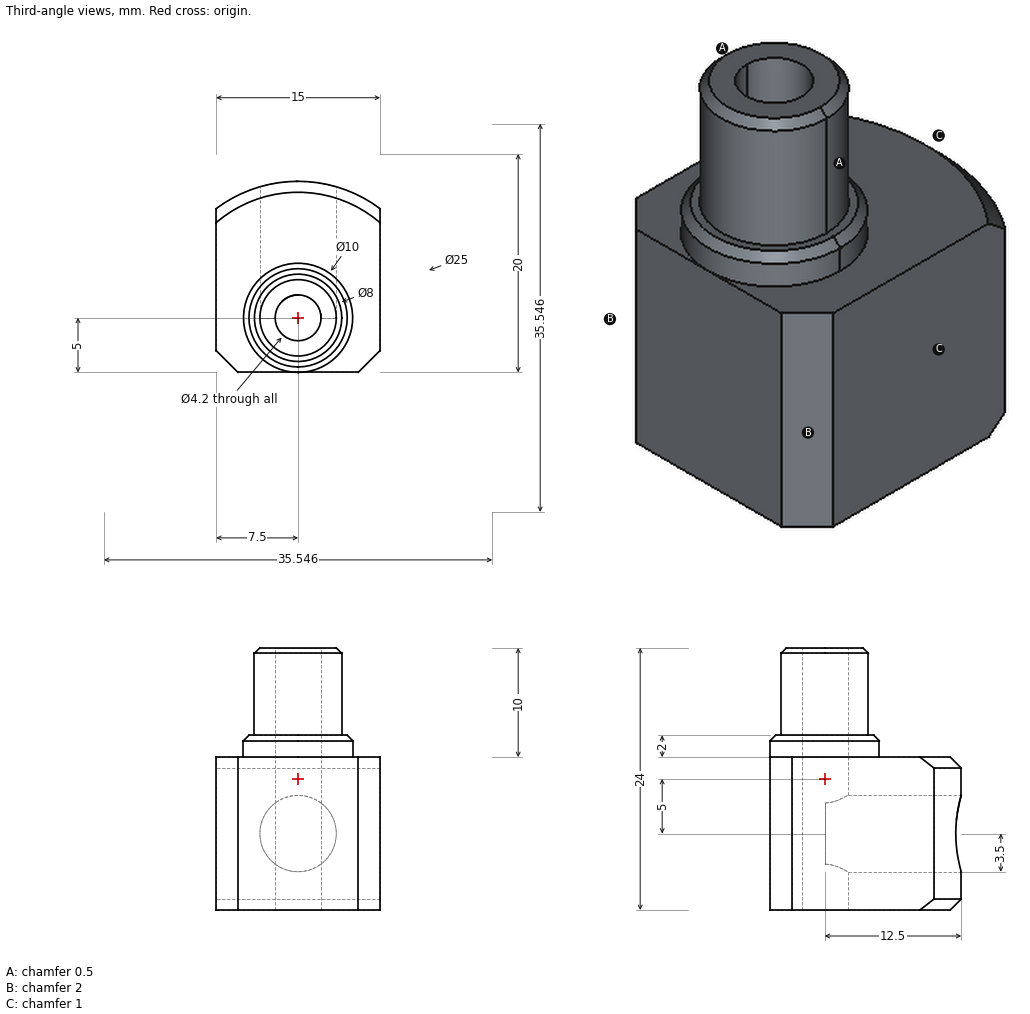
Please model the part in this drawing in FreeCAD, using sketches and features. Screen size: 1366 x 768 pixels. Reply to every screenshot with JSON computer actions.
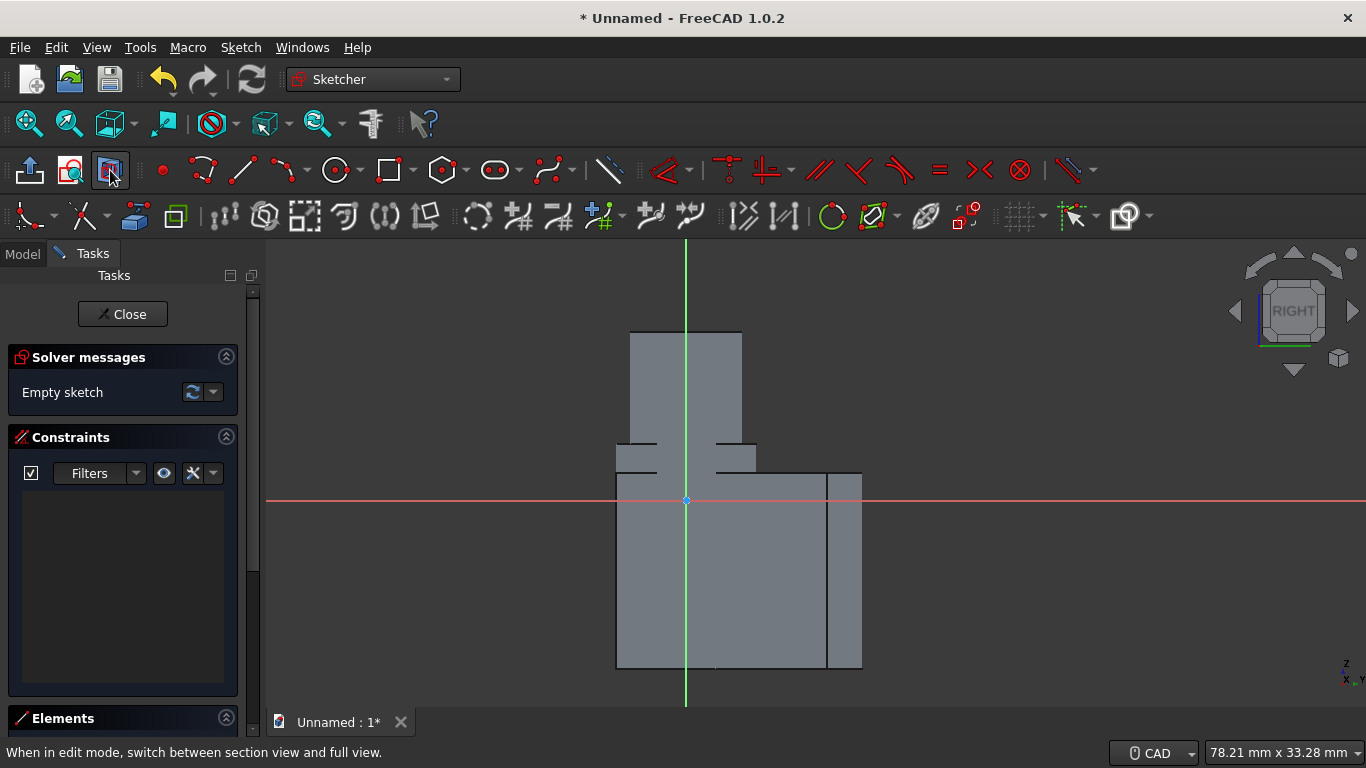
{"action": "scroll", "coordinate": [860, 632], "scroll_direction": "up", "scroll_amount": 4}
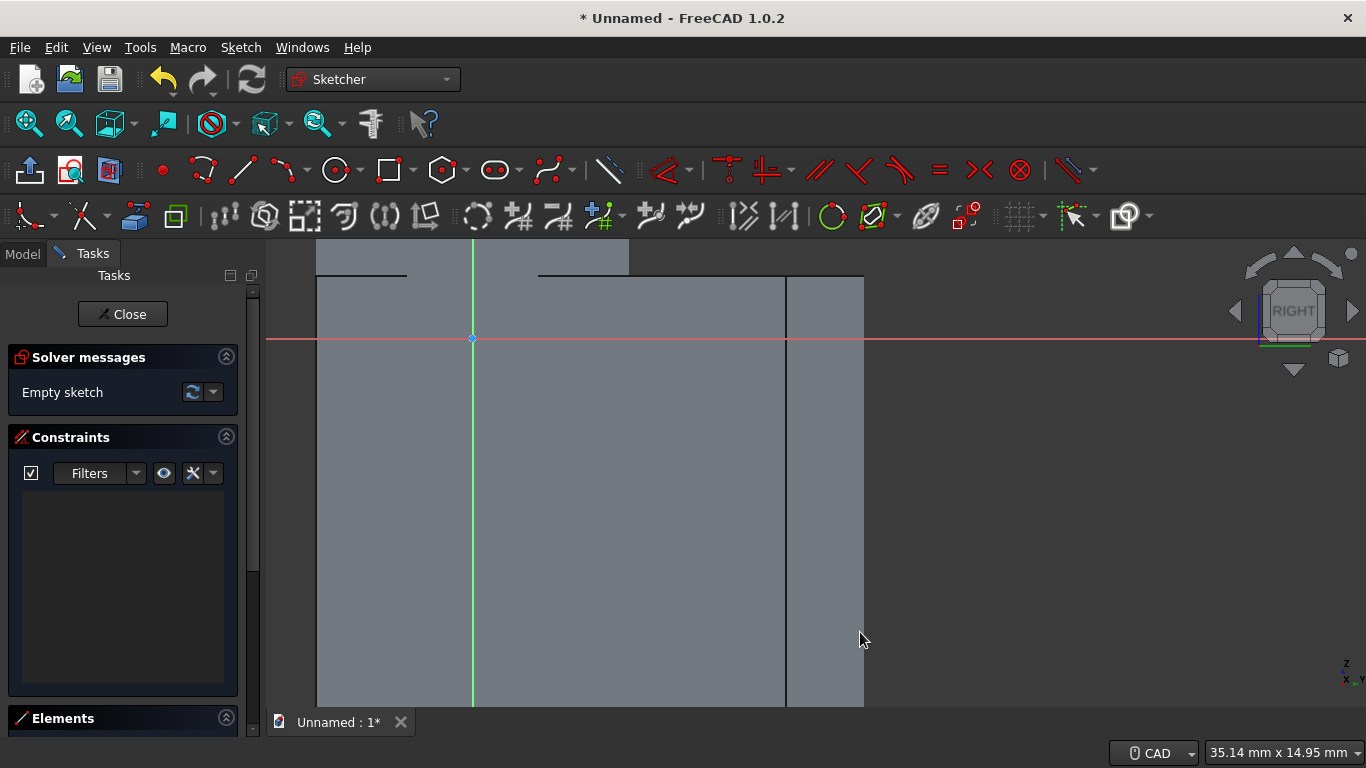
{"action": "left_click", "coordinate": [390, 170]}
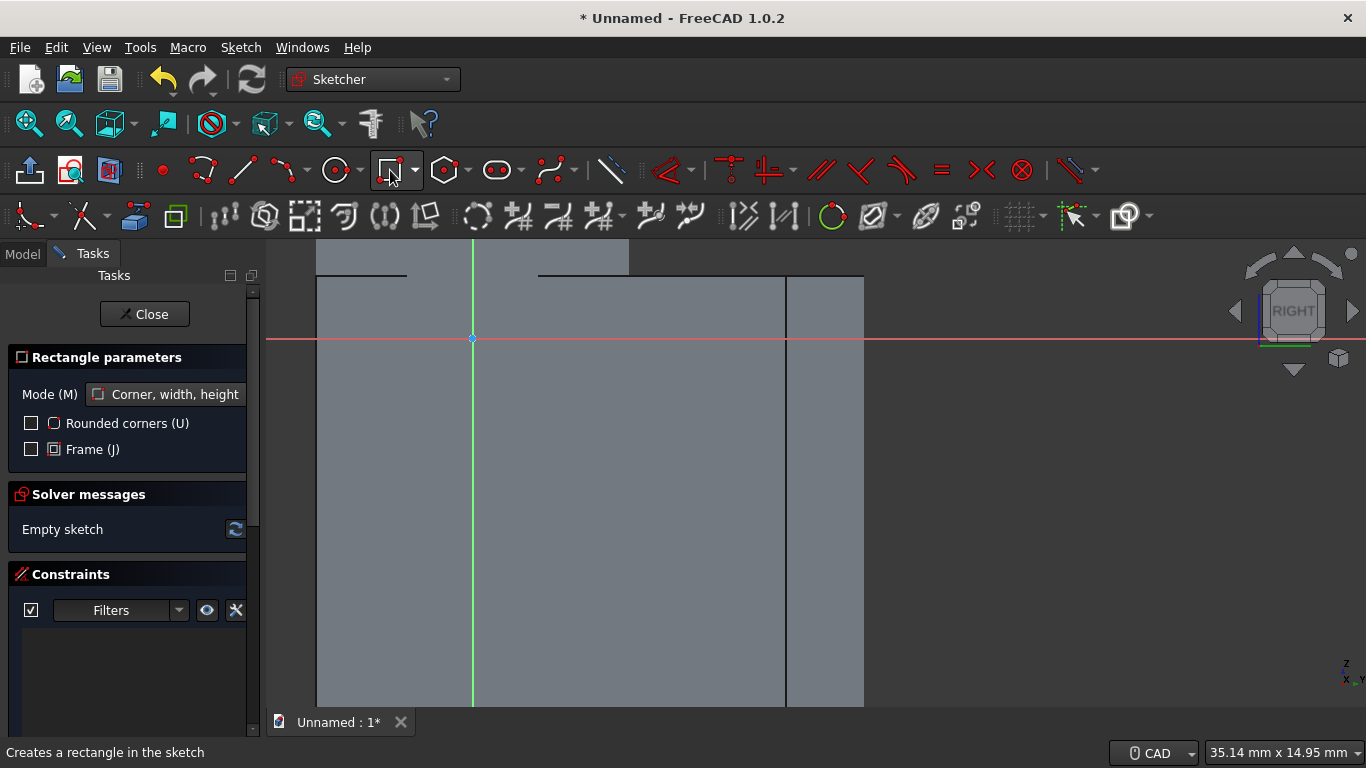
{"action": "left_click", "coordinate": [473, 495]}
{"action": "mouse_move", "coordinate": [864, 605]}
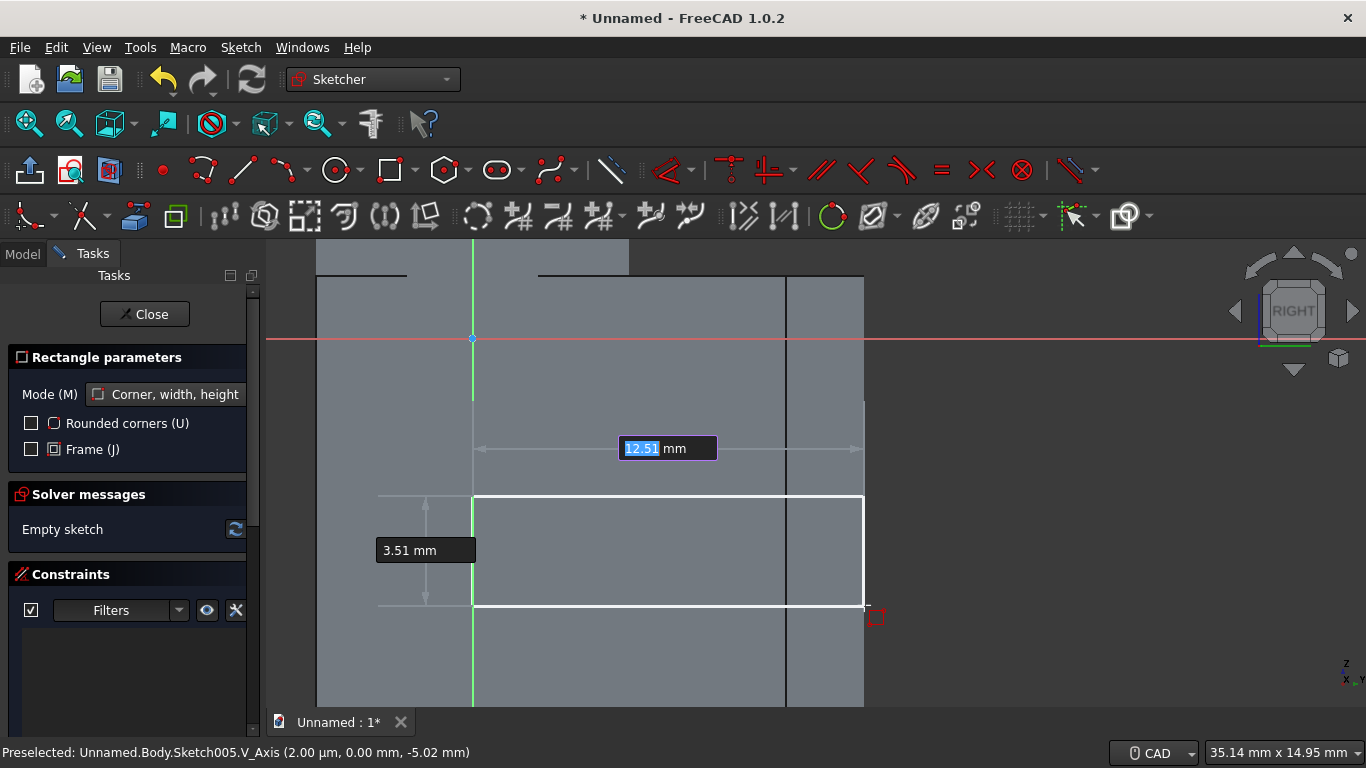
{"action": "type", "text": "12.5"}
{"action": "key", "text": "Tab"}
{"action": "type", "text": "3.5"}
{"action": "key", "text": "Return"}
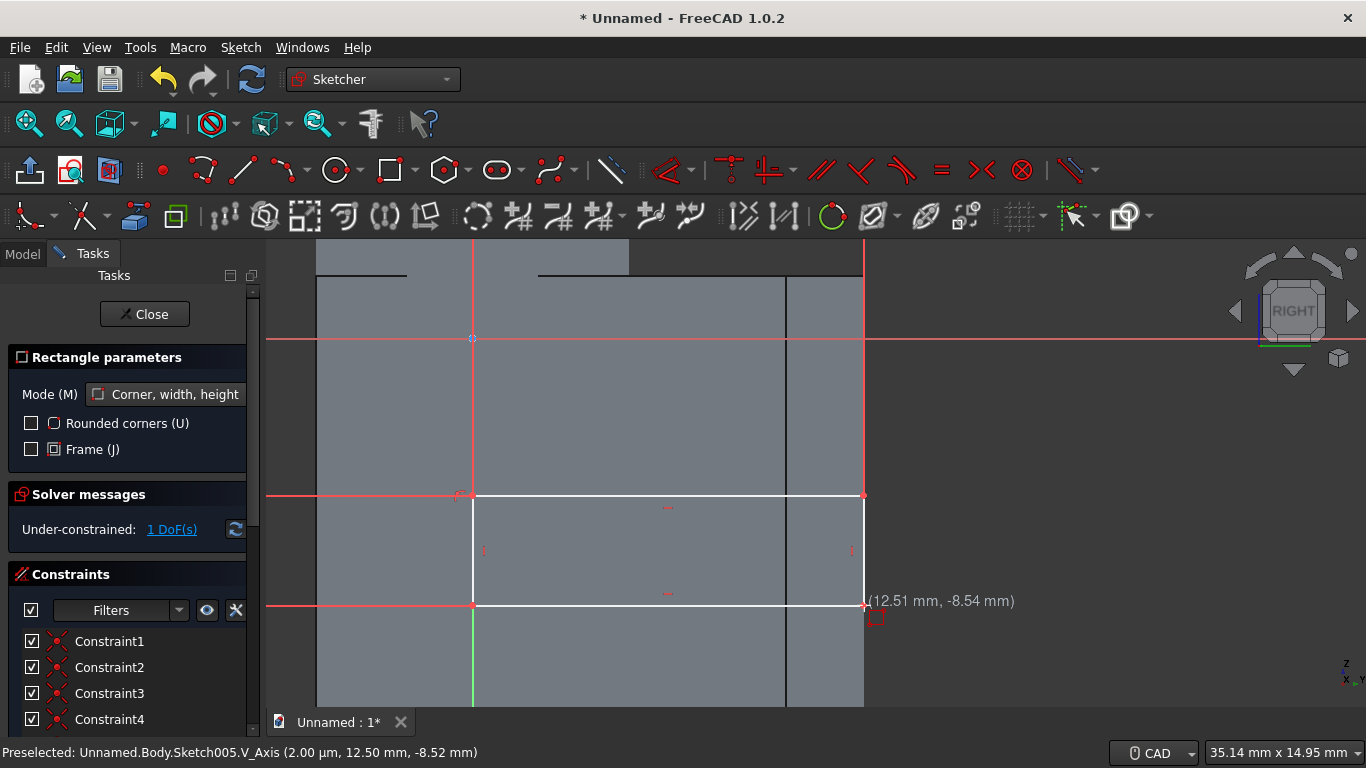
{"action": "key", "text": "g l"}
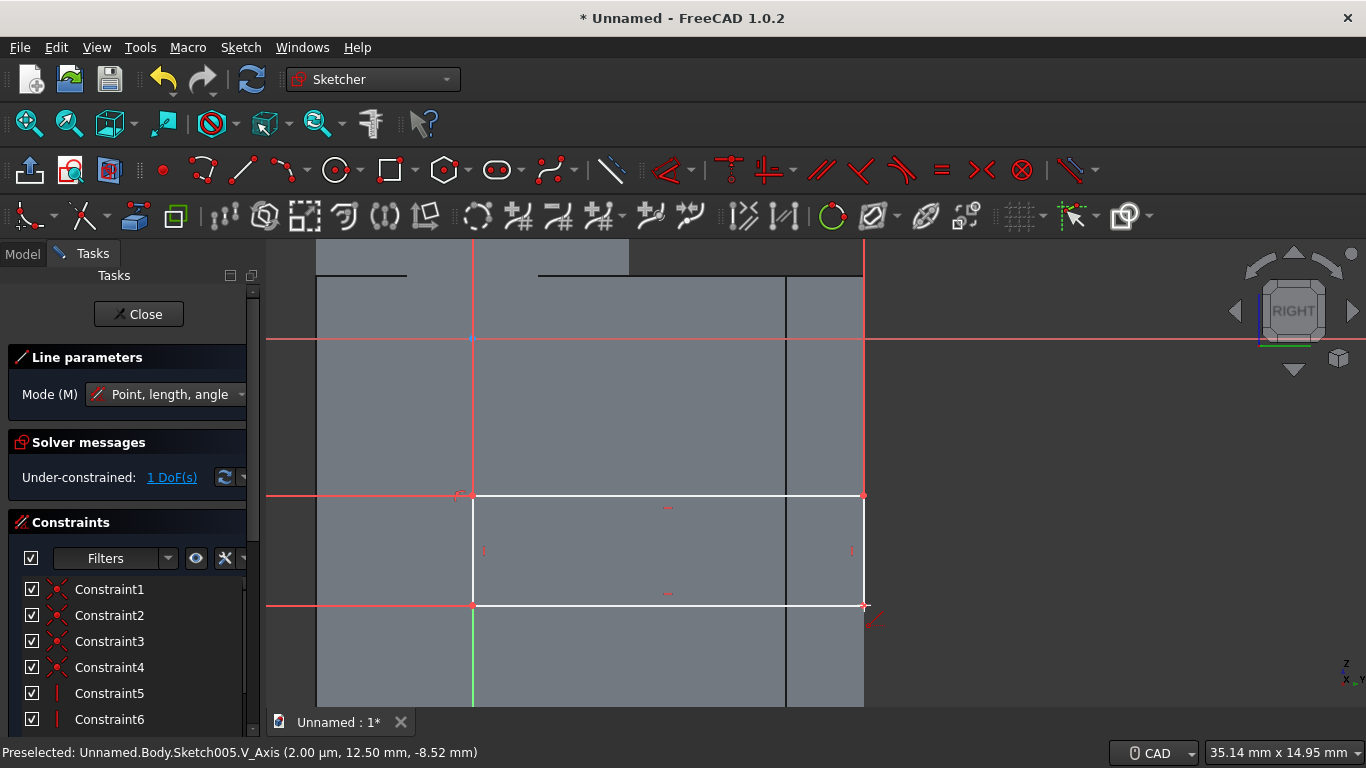
{"action": "left_click", "coordinate": [903, 495]}
{"action": "left_click", "coordinate": [1020, 495]}
{"action": "key", "text": "Escape"}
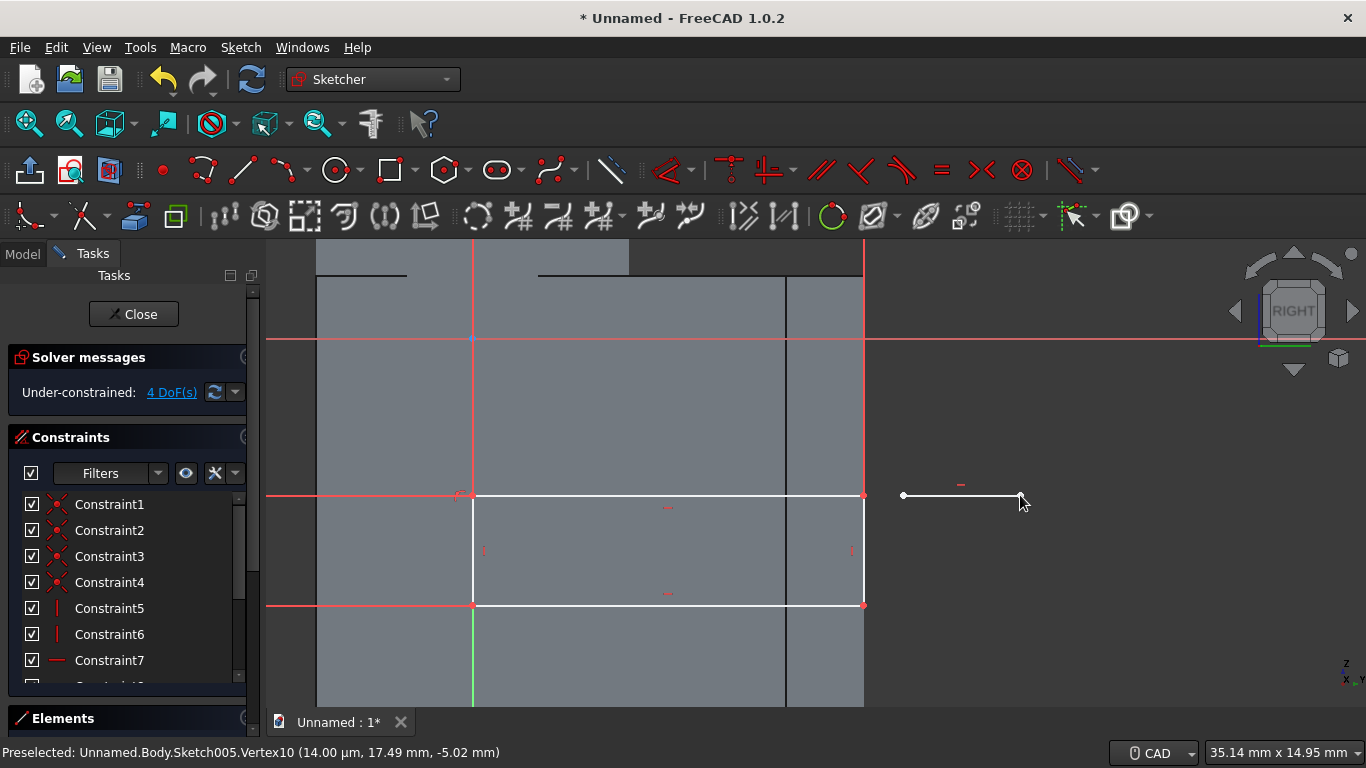
{"action": "left_click", "coordinate": [938, 496]}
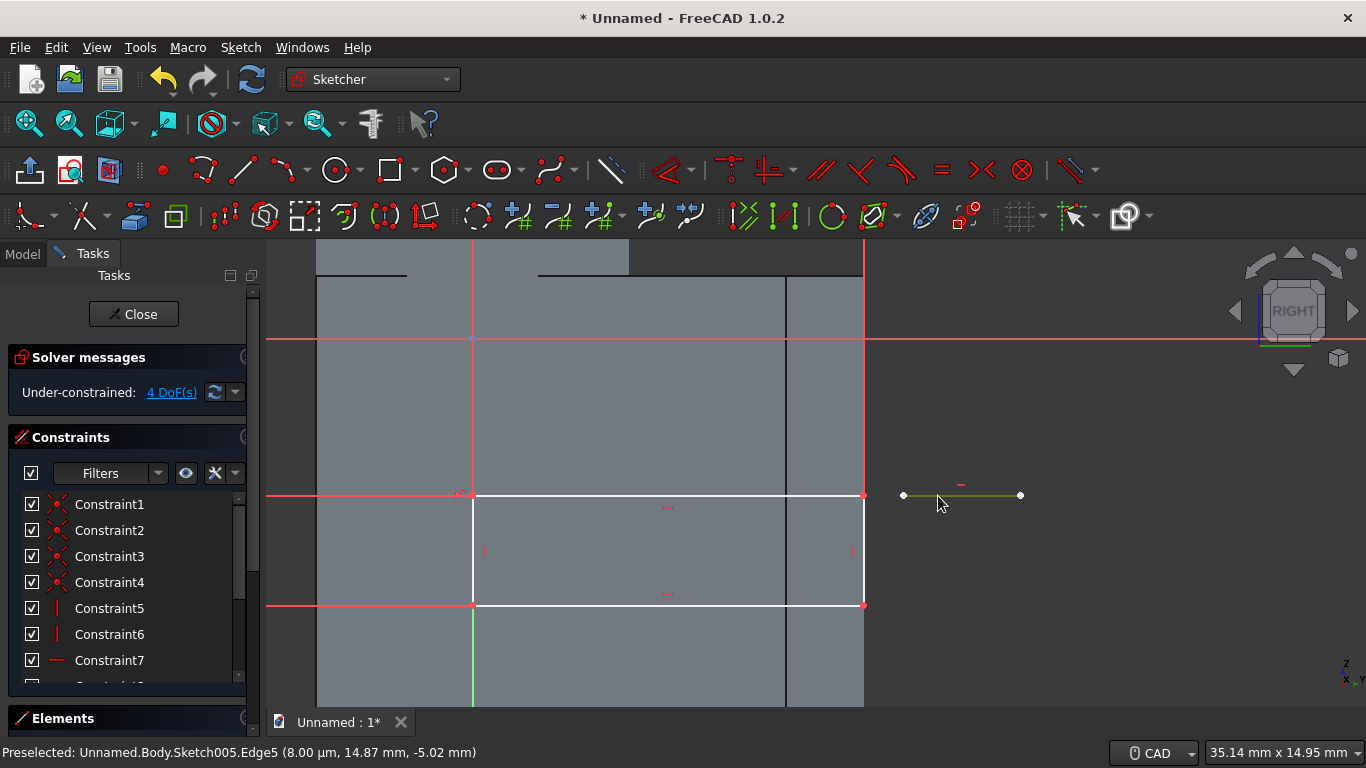
{"action": "left_click", "coordinate": [612, 170]}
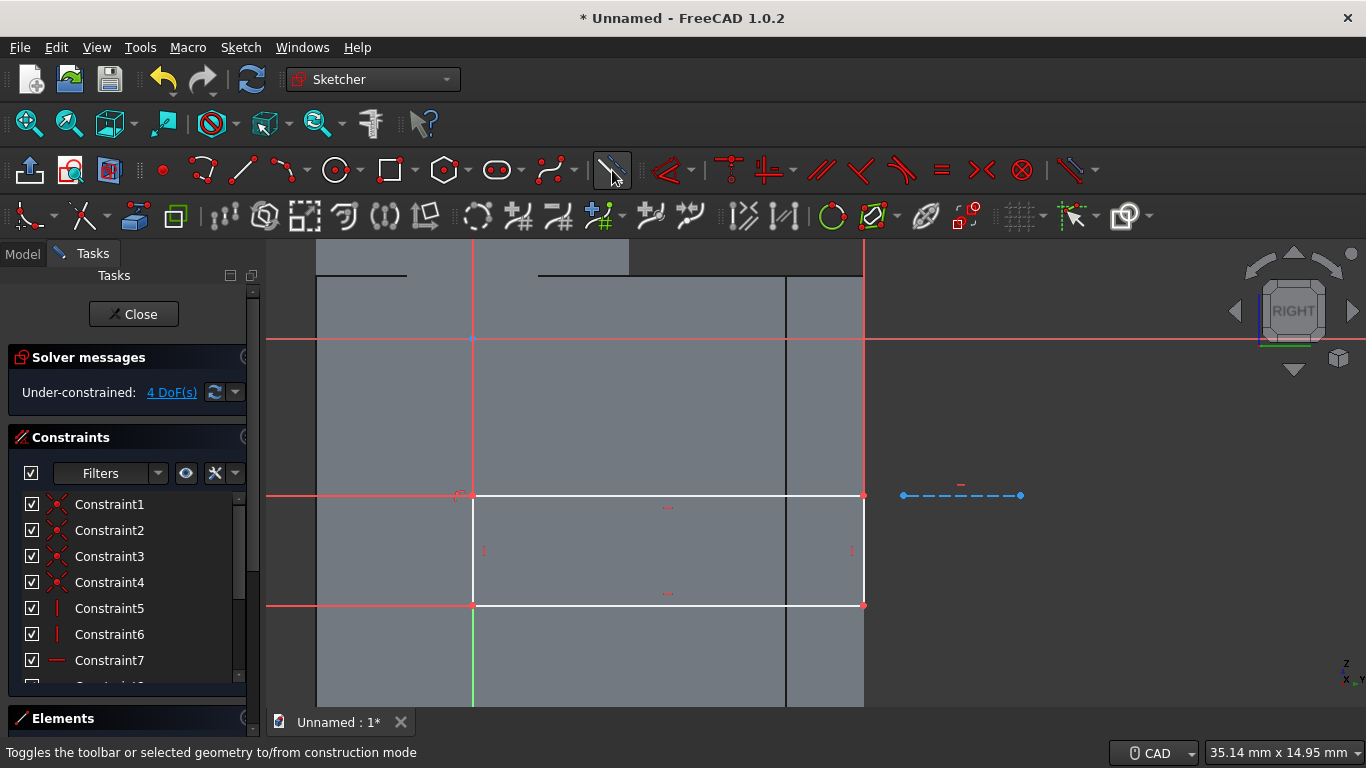
{"action": "key", "text": "d"}